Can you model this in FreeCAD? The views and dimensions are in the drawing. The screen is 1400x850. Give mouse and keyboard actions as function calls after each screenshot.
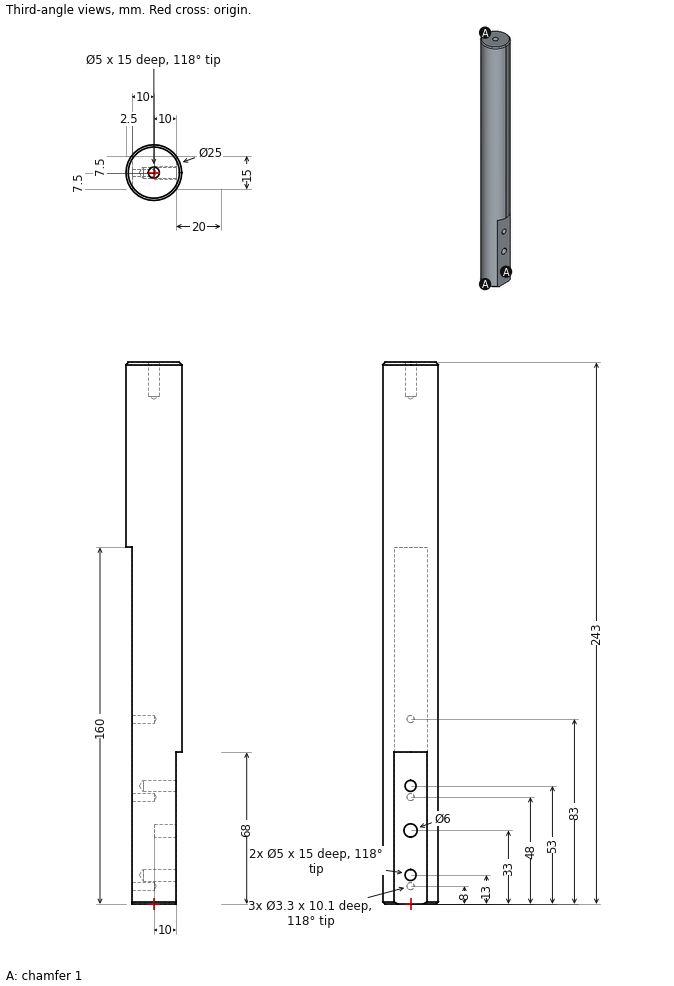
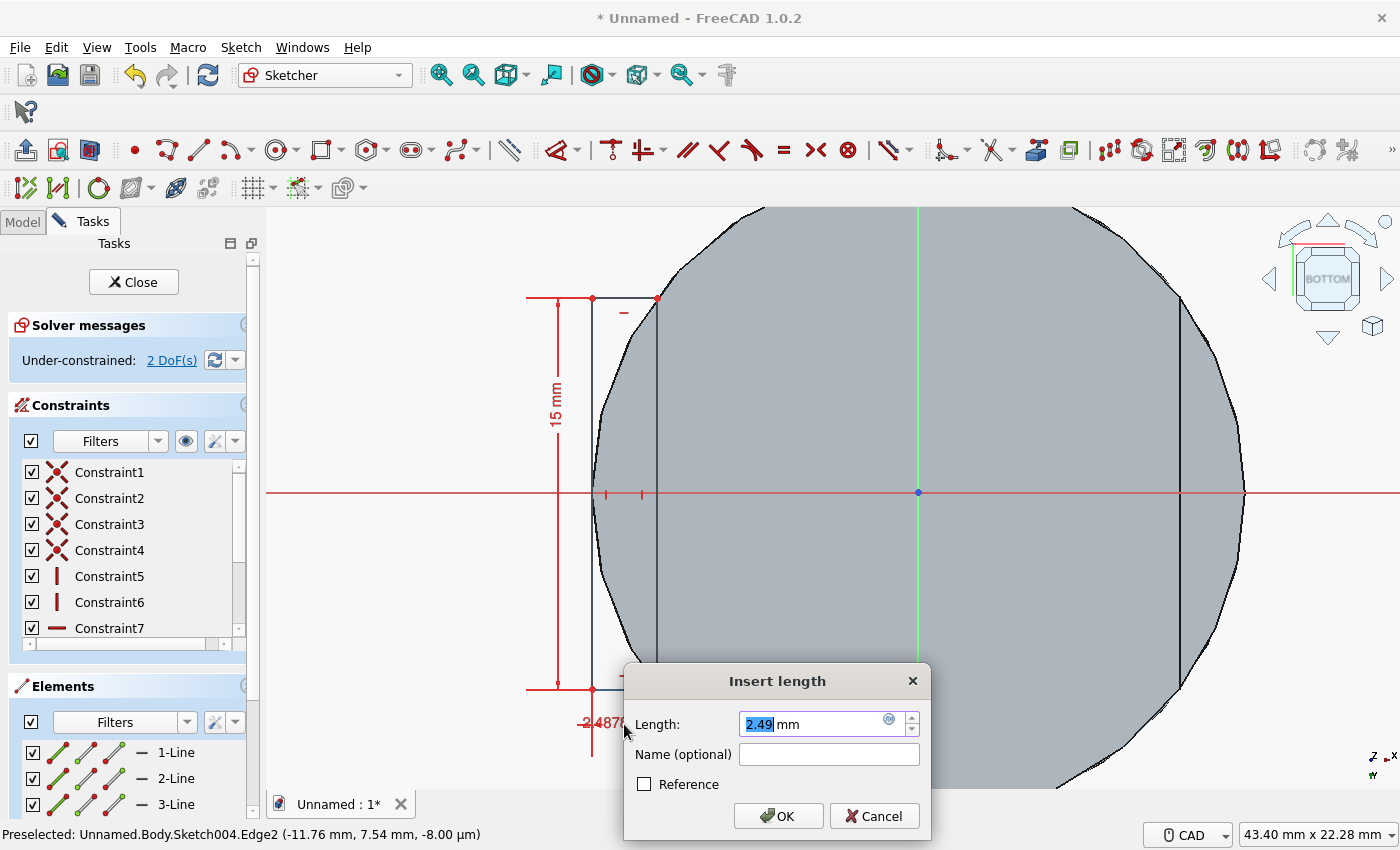
text(2.5)
key(Return)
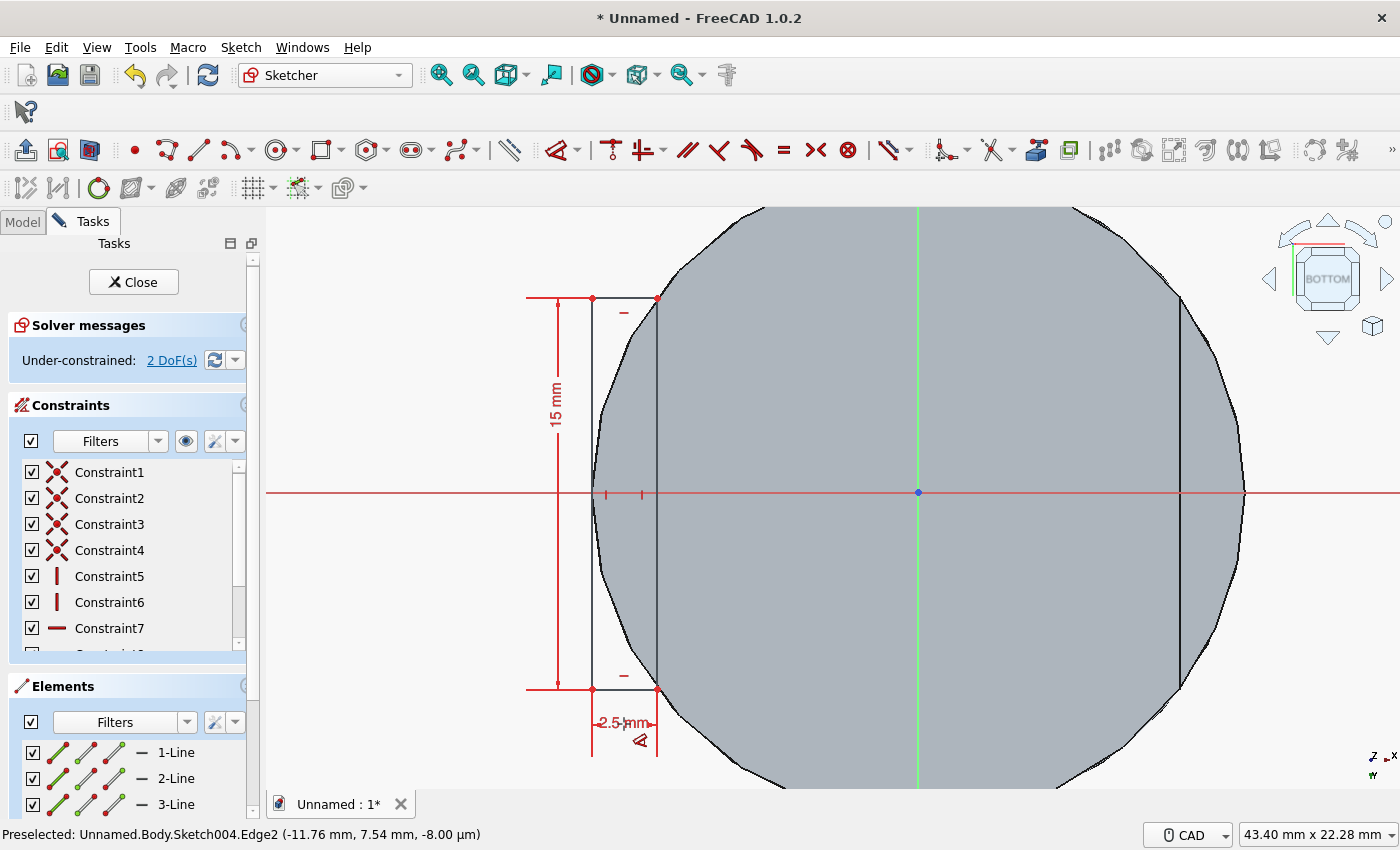
click(657, 690)
click(788, 724)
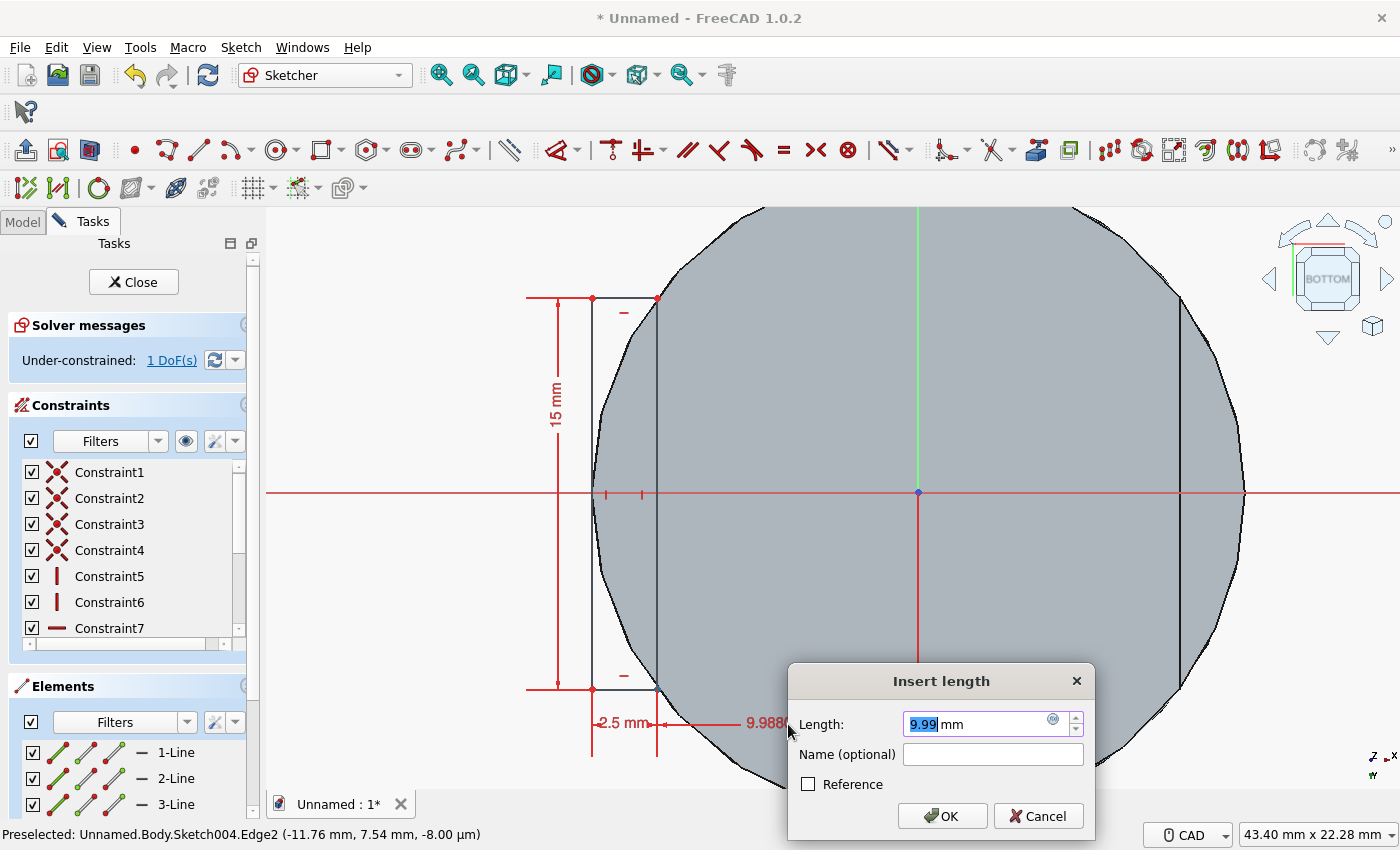
text(10)
key(Return)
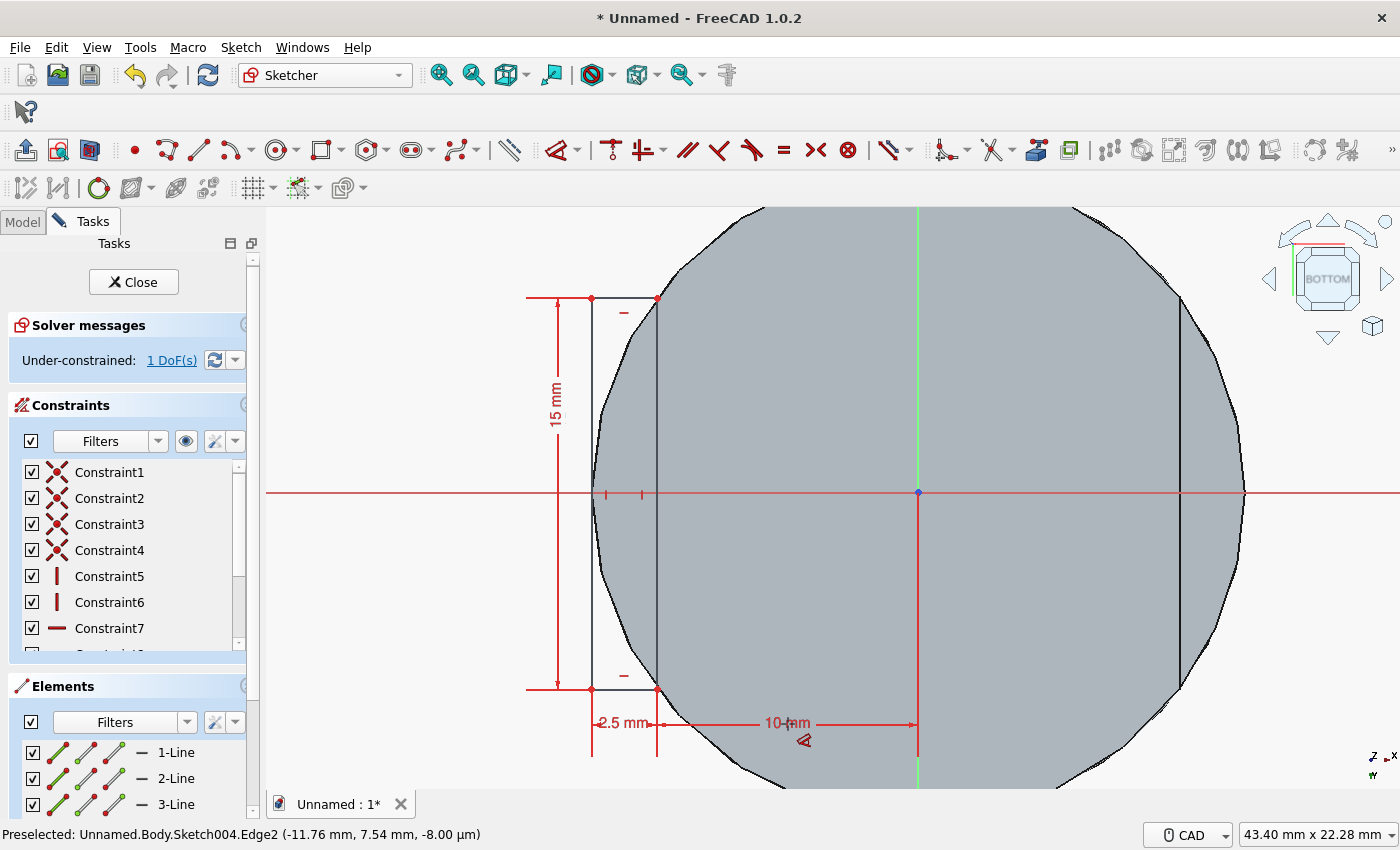
click(592, 298)
click(952, 396)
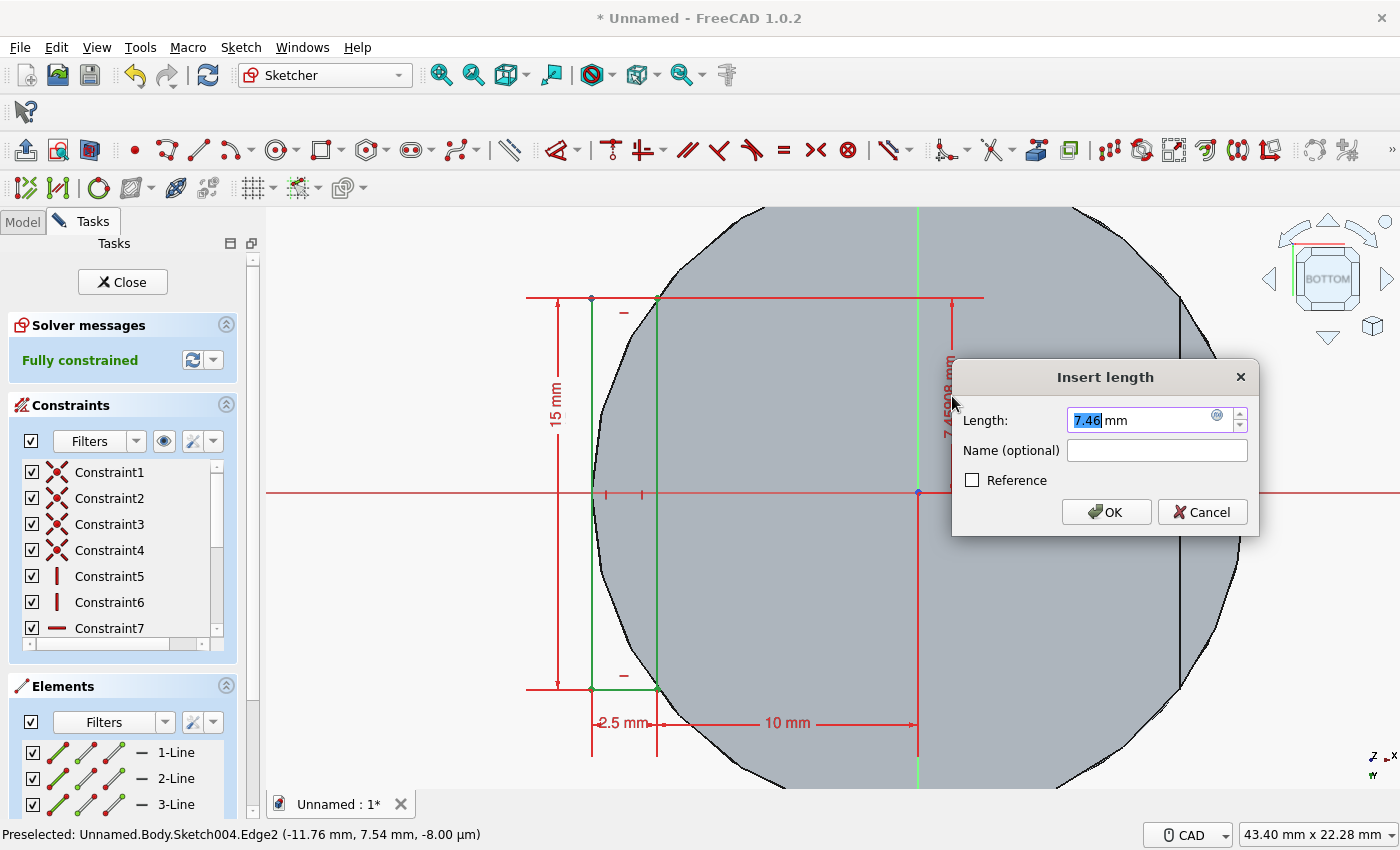
text(7.5)
key(Return)
key(Escape)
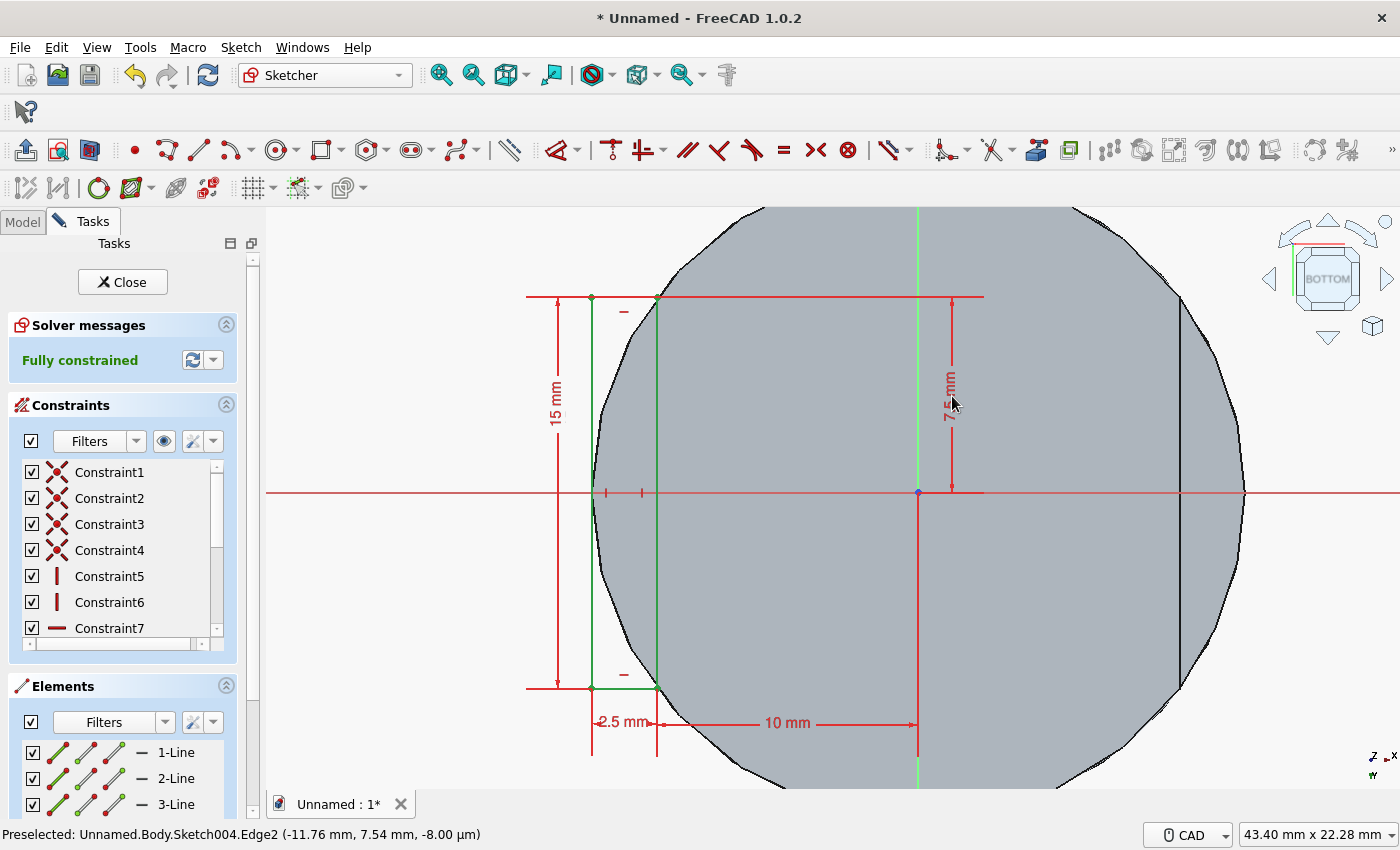
click(123, 282)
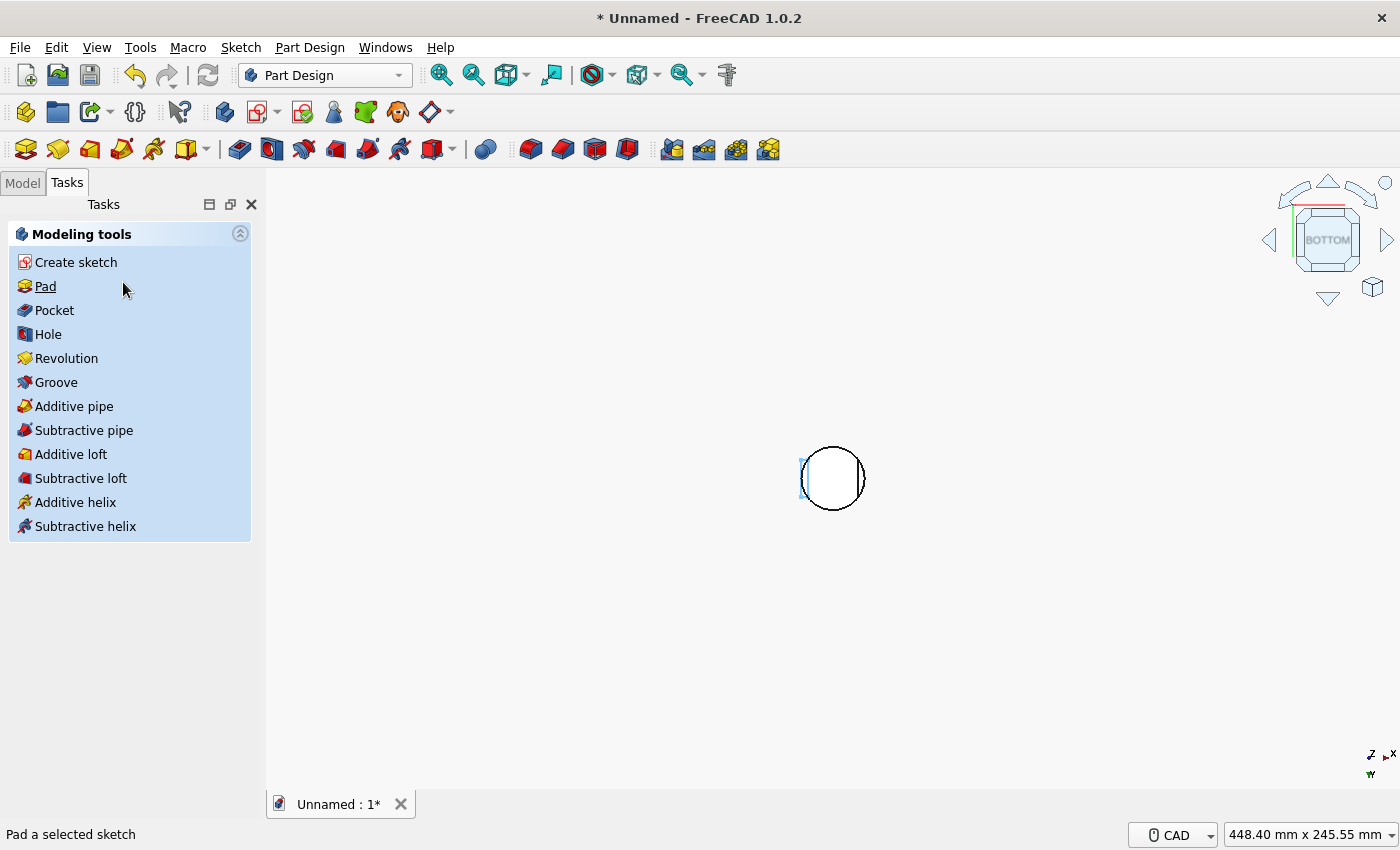
click(240, 150)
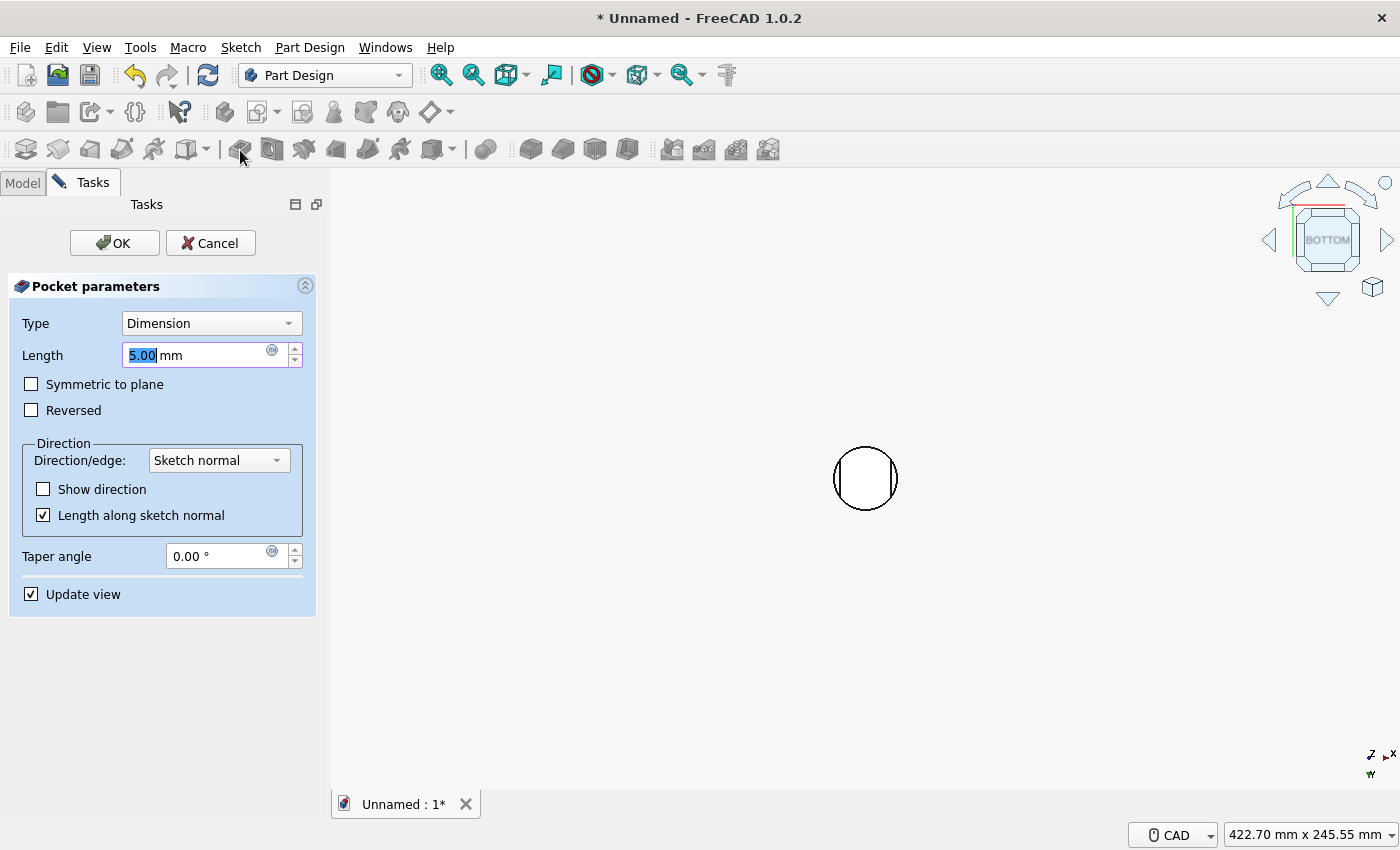
text(160)
key(Tab)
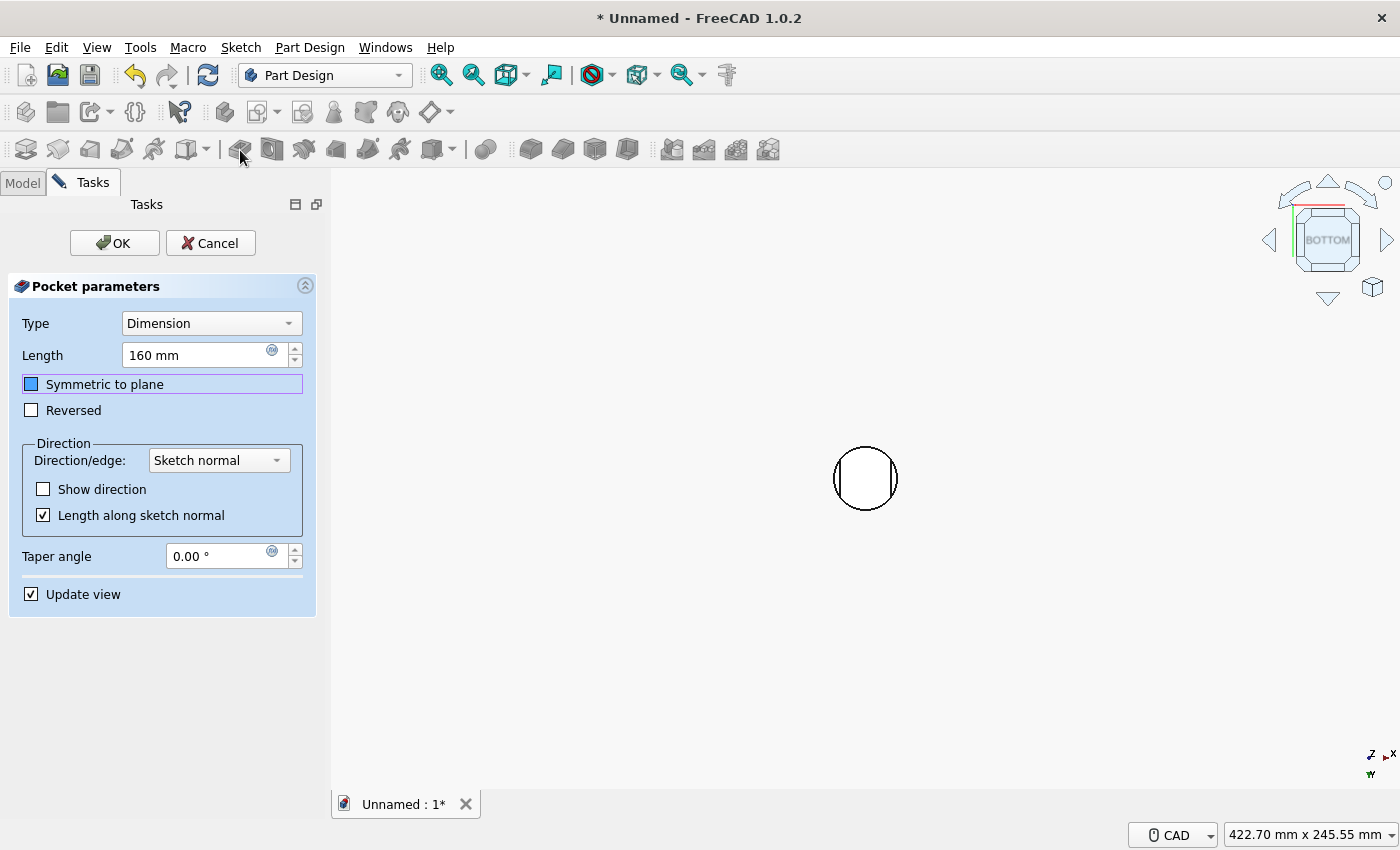
click(115, 243)